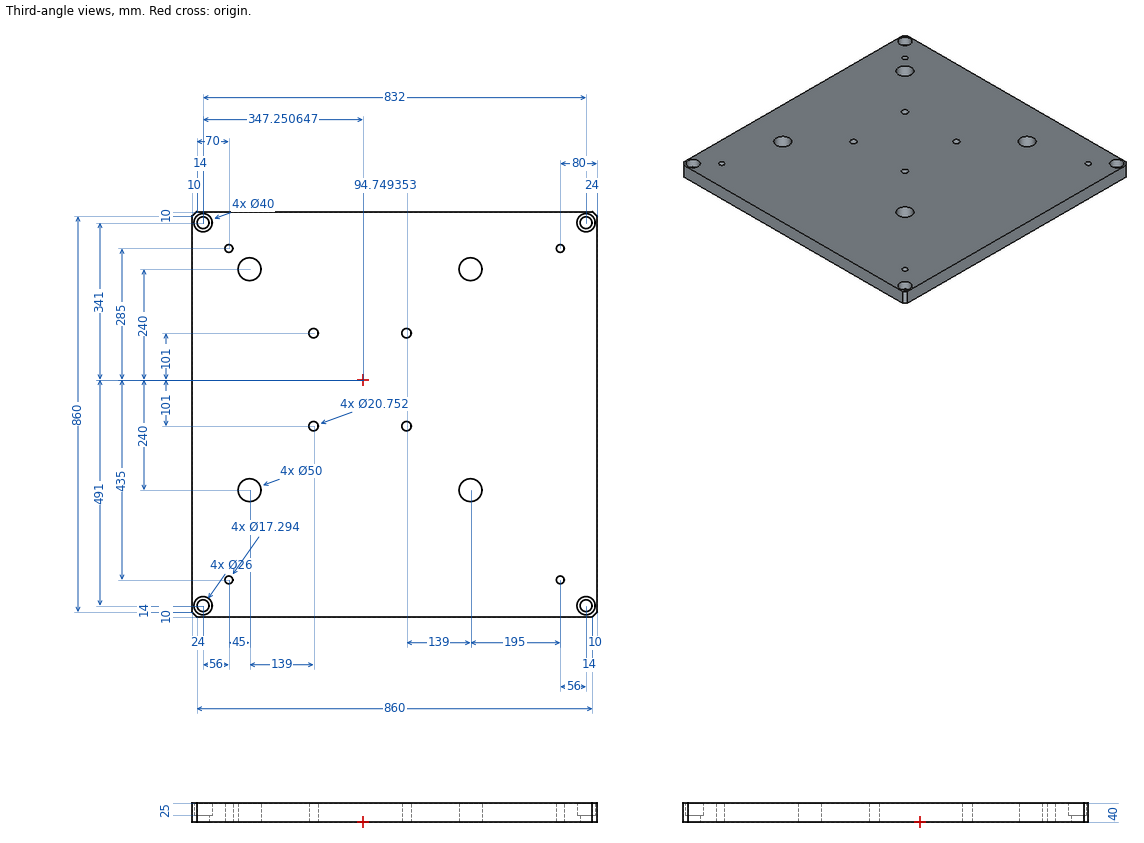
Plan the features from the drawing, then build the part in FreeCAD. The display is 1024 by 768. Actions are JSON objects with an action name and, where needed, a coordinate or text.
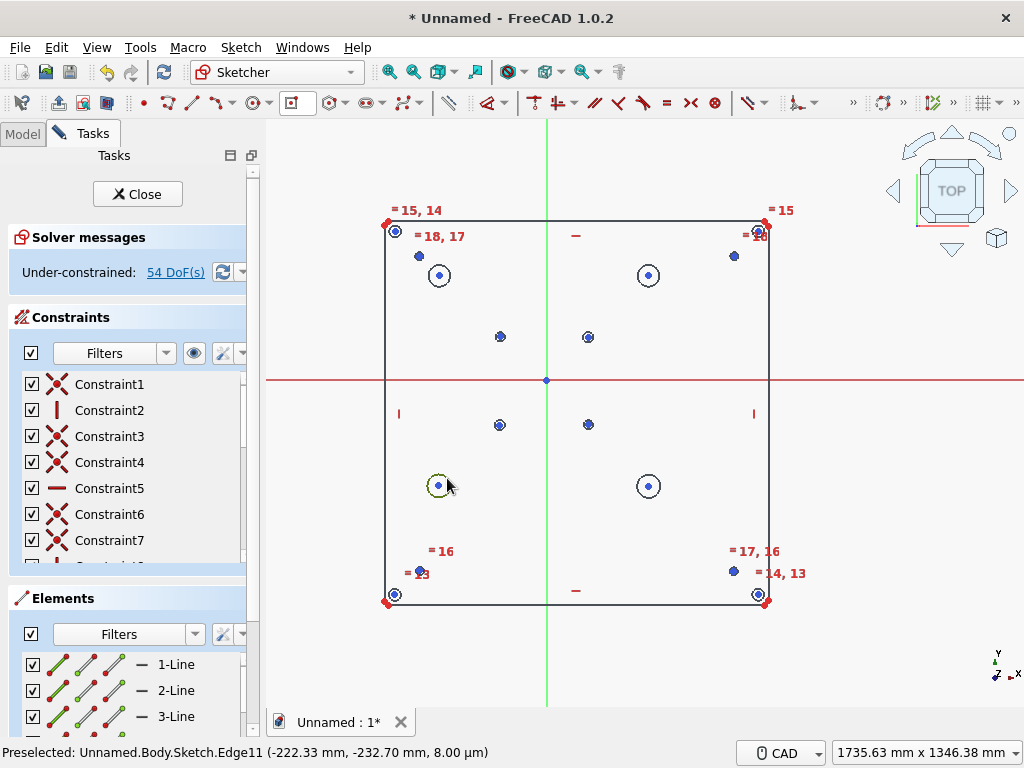
{"action": "left_click", "coordinate": [657, 478]}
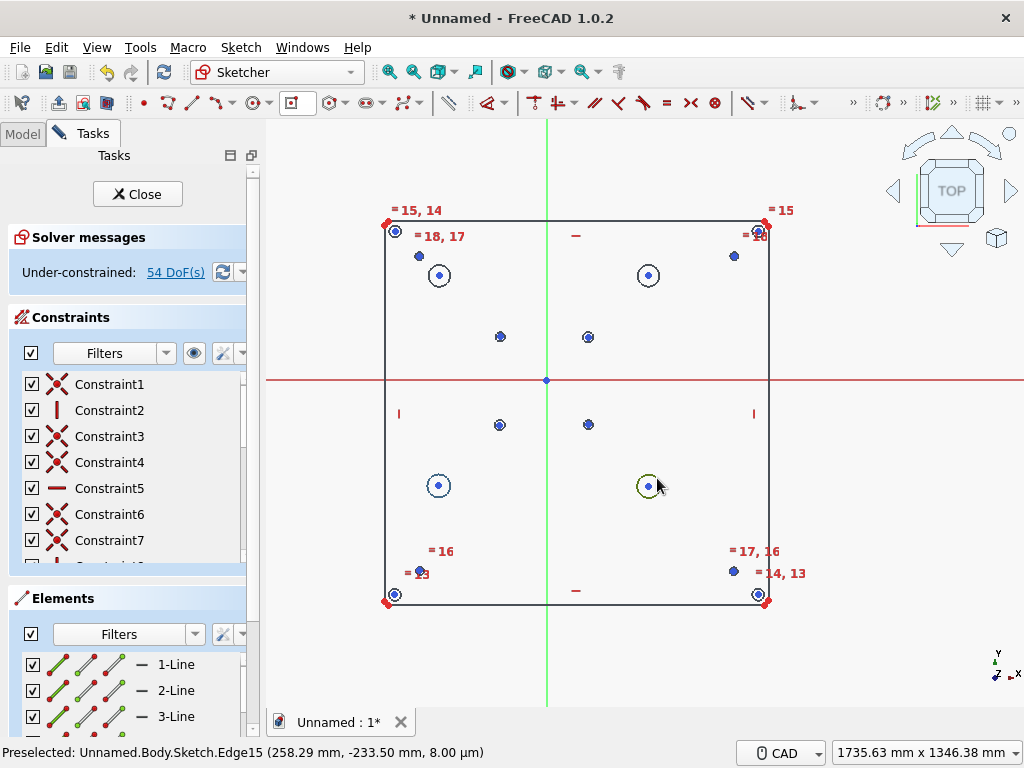
{"action": "scroll", "coordinate": [447, 268], "scroll_direction": "up", "scroll_amount": 2}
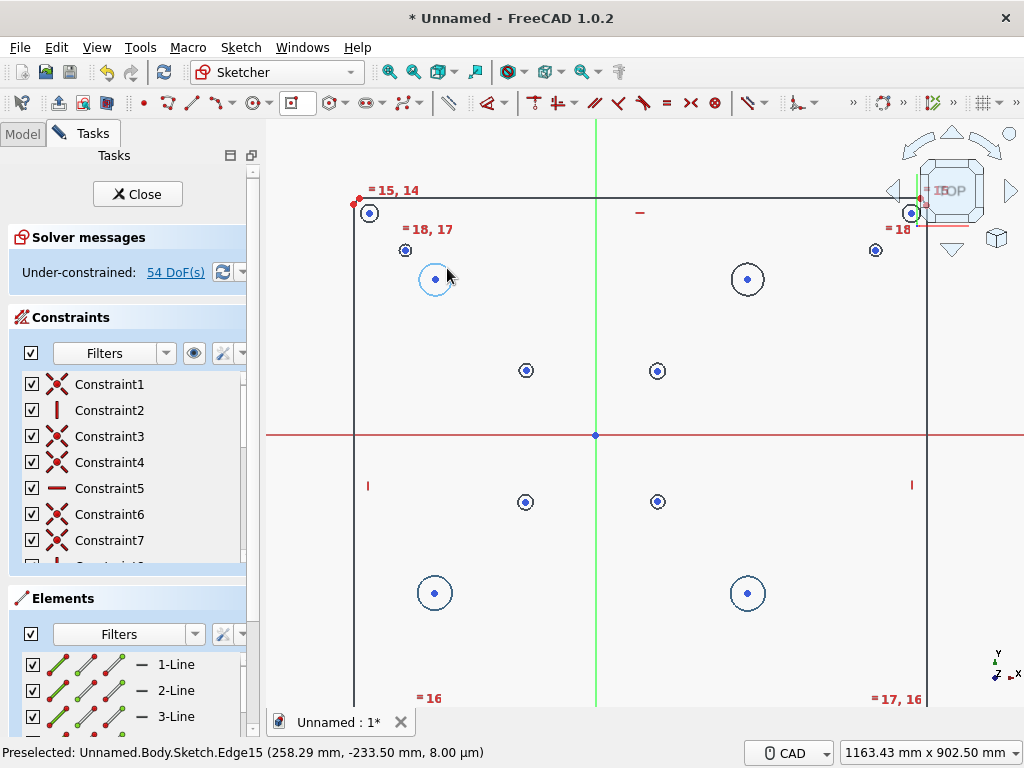
{"action": "left_click", "coordinate": [447, 268]}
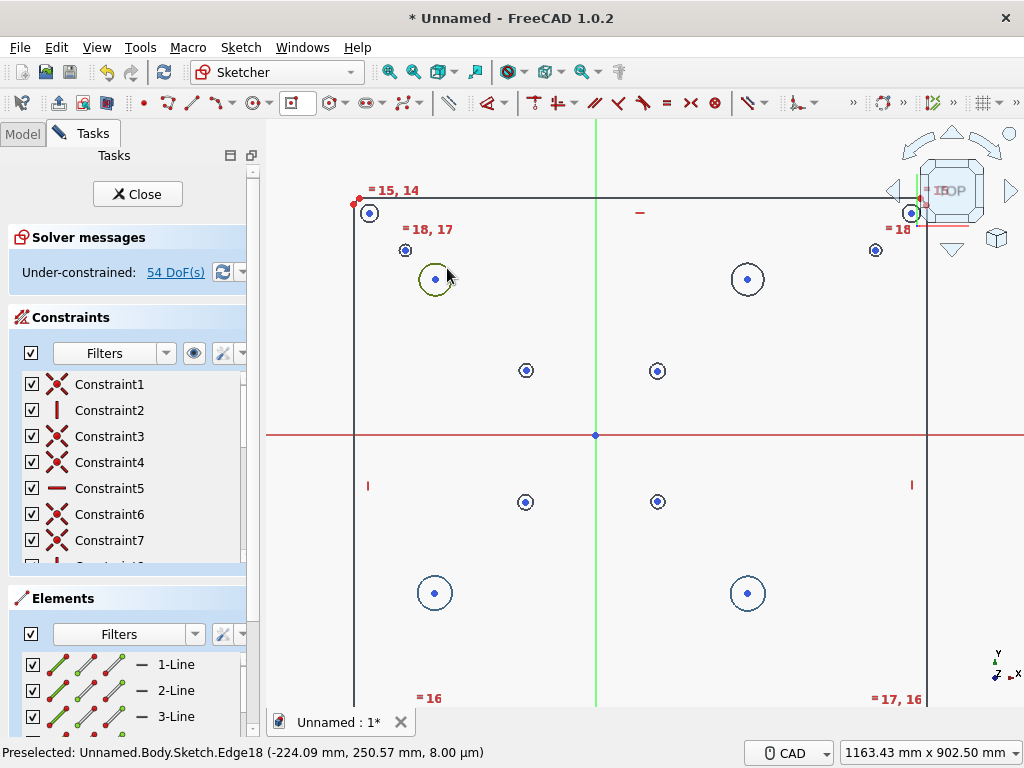
{"action": "left_click", "coordinate": [759, 268]}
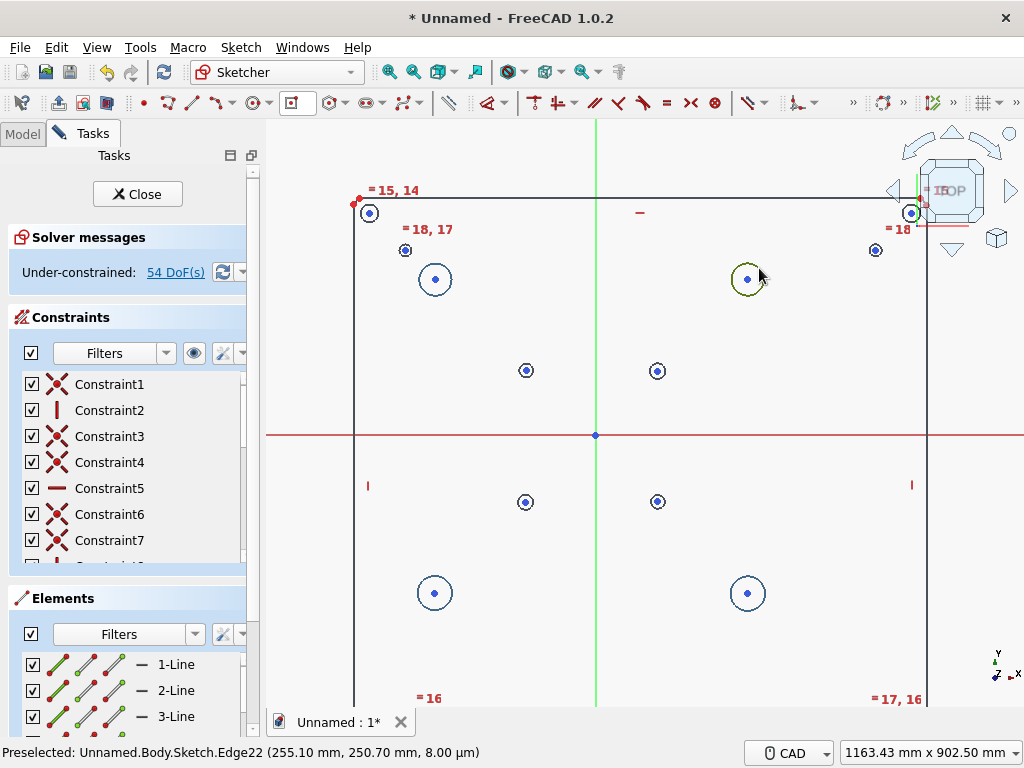
{"action": "left_click", "coordinate": [668, 104]}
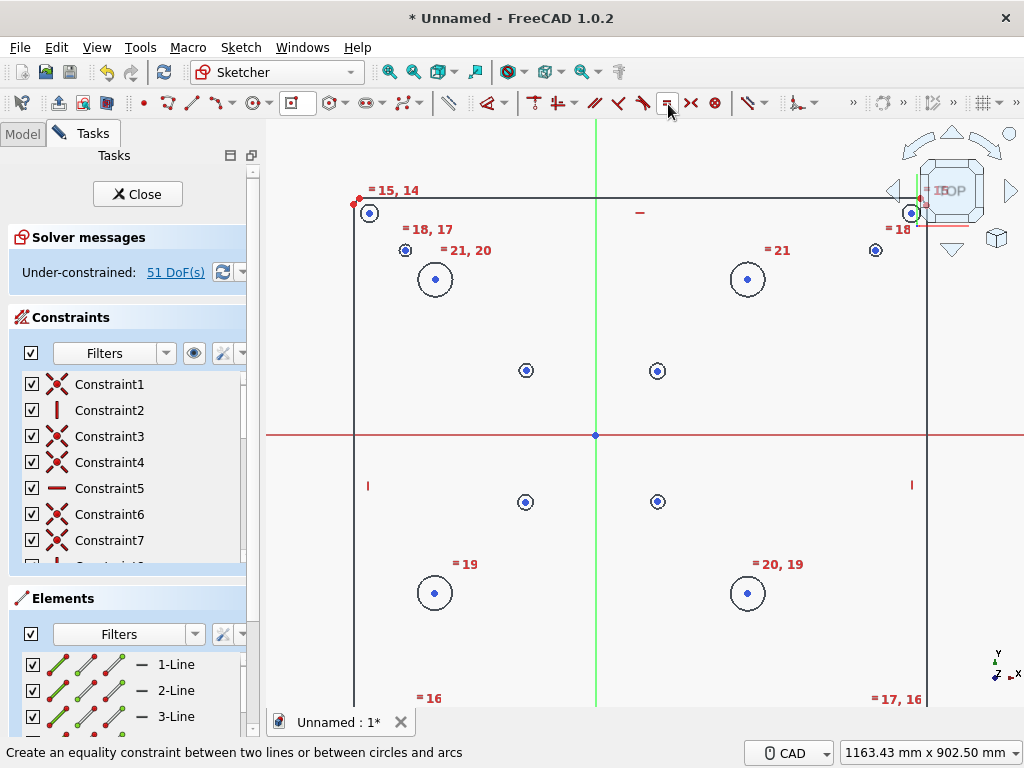
{"action": "scroll", "coordinate": [531, 508], "scroll_direction": "up", "scroll_amount": 4}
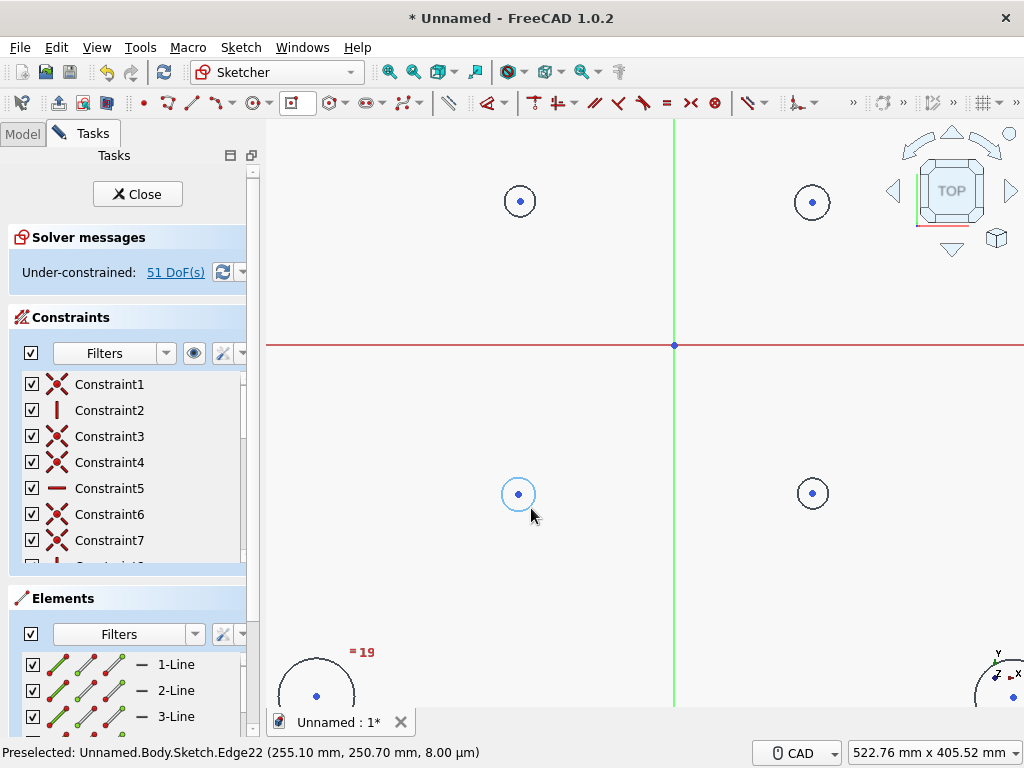
{"action": "left_click", "coordinate": [530, 506]}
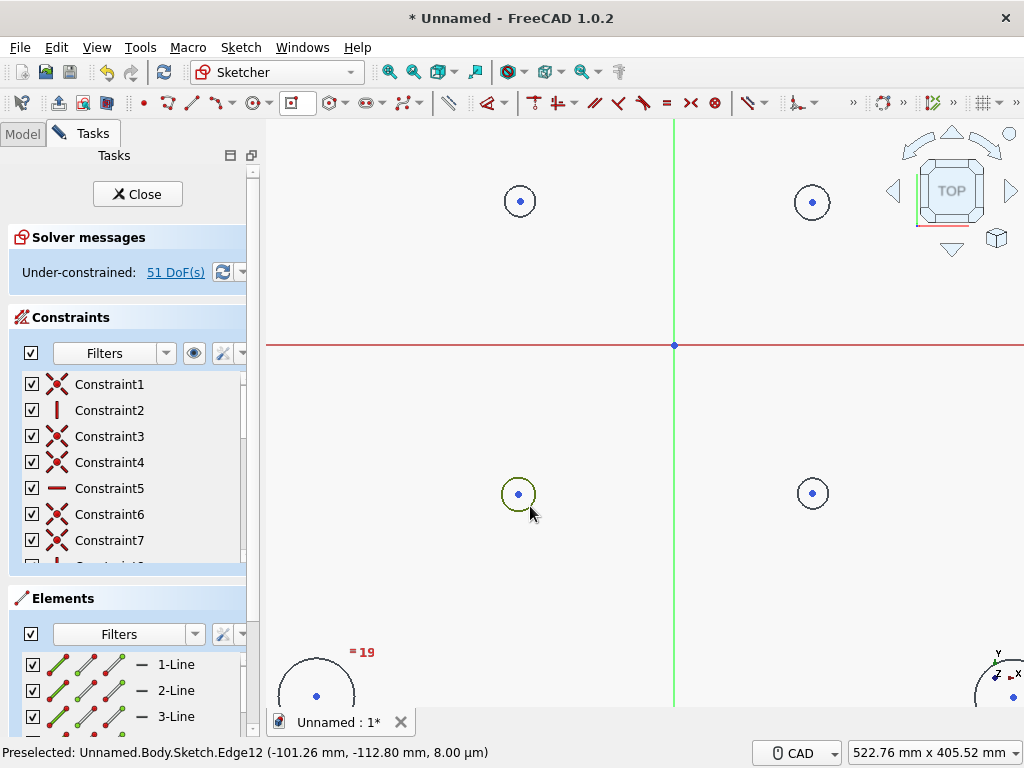
{"action": "left_click", "coordinate": [824, 483]}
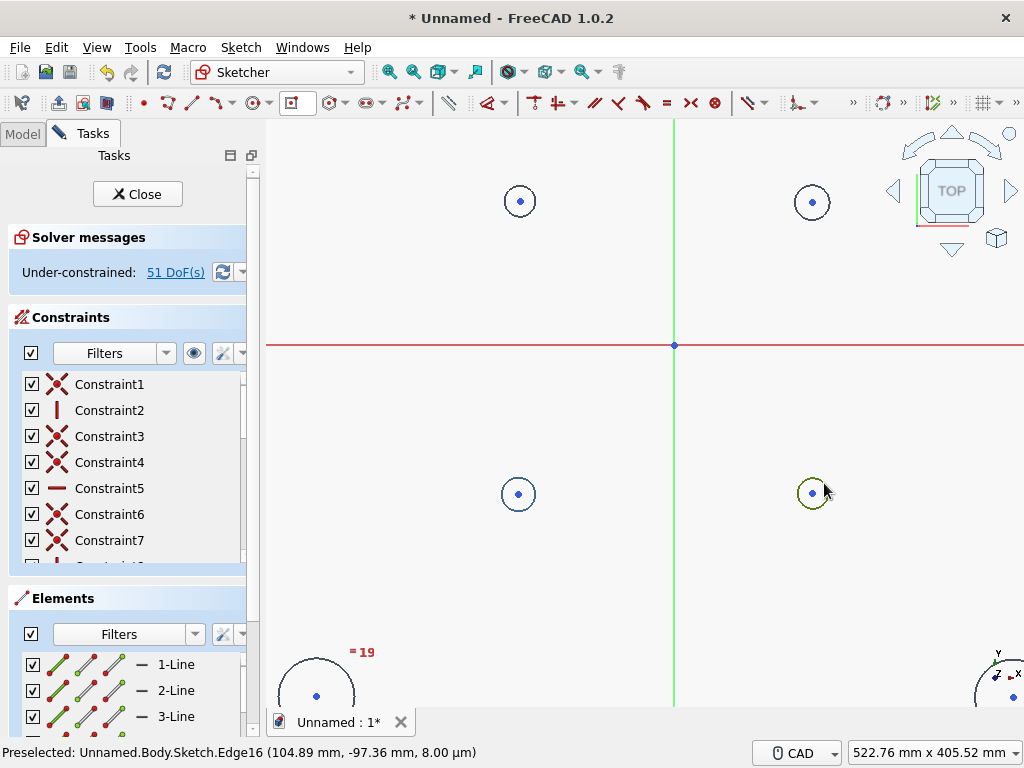
{"action": "left_click", "coordinate": [531, 190]}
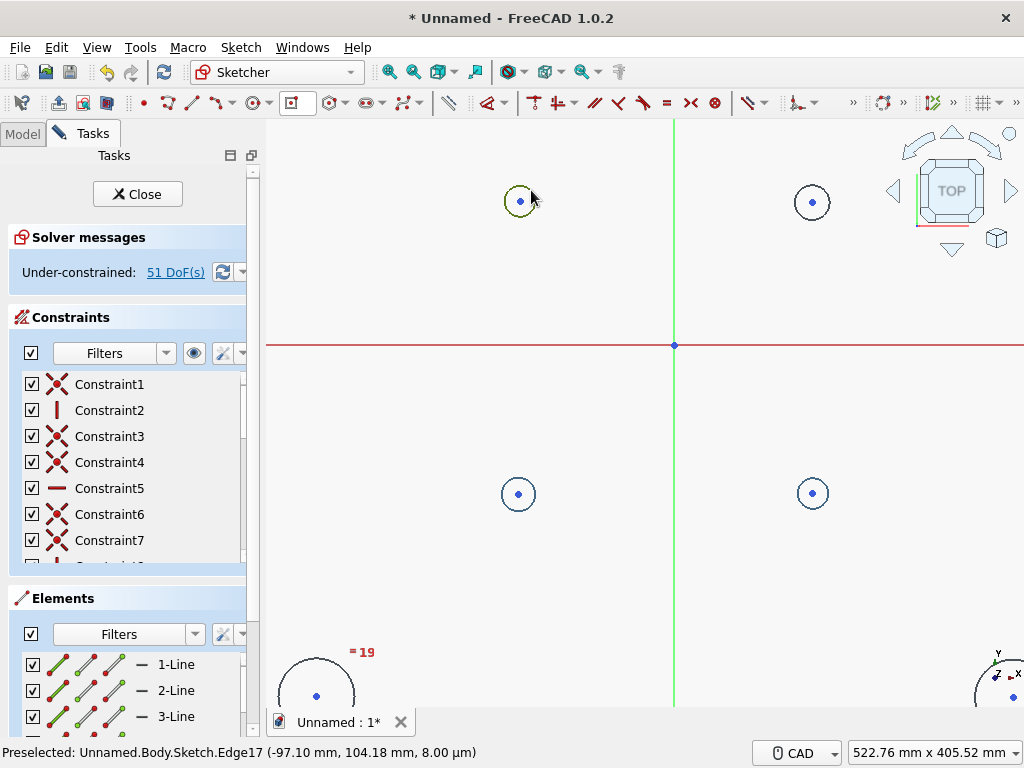
{"action": "left_click", "coordinate": [824, 190]}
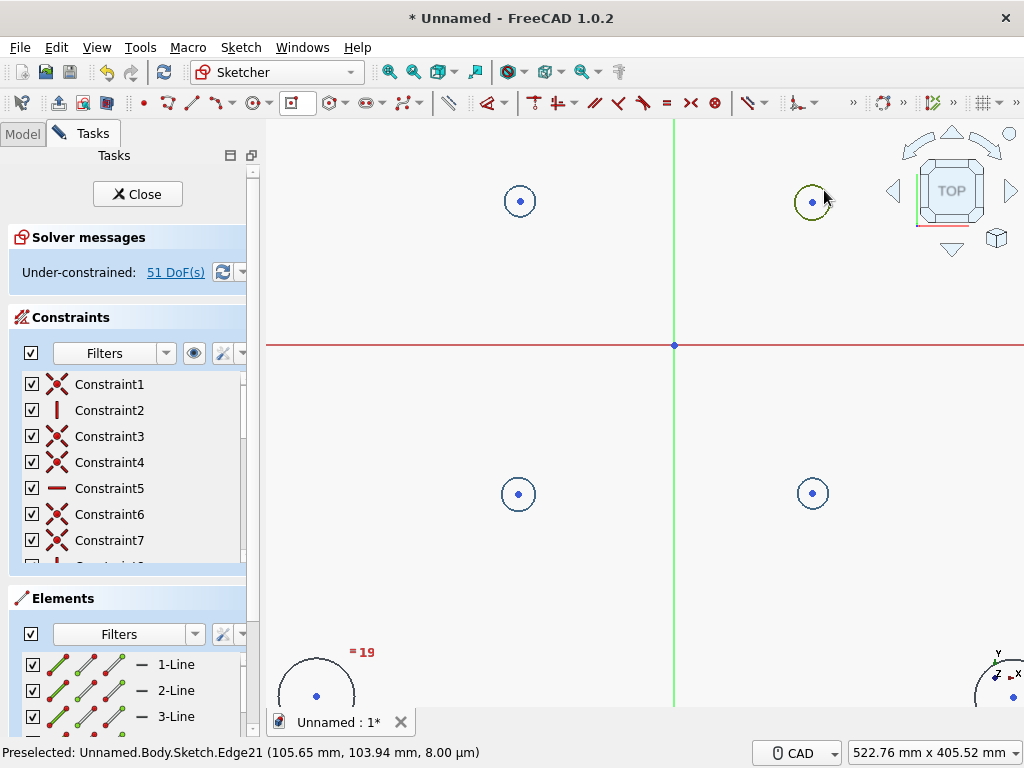
{"action": "key", "text": "e"}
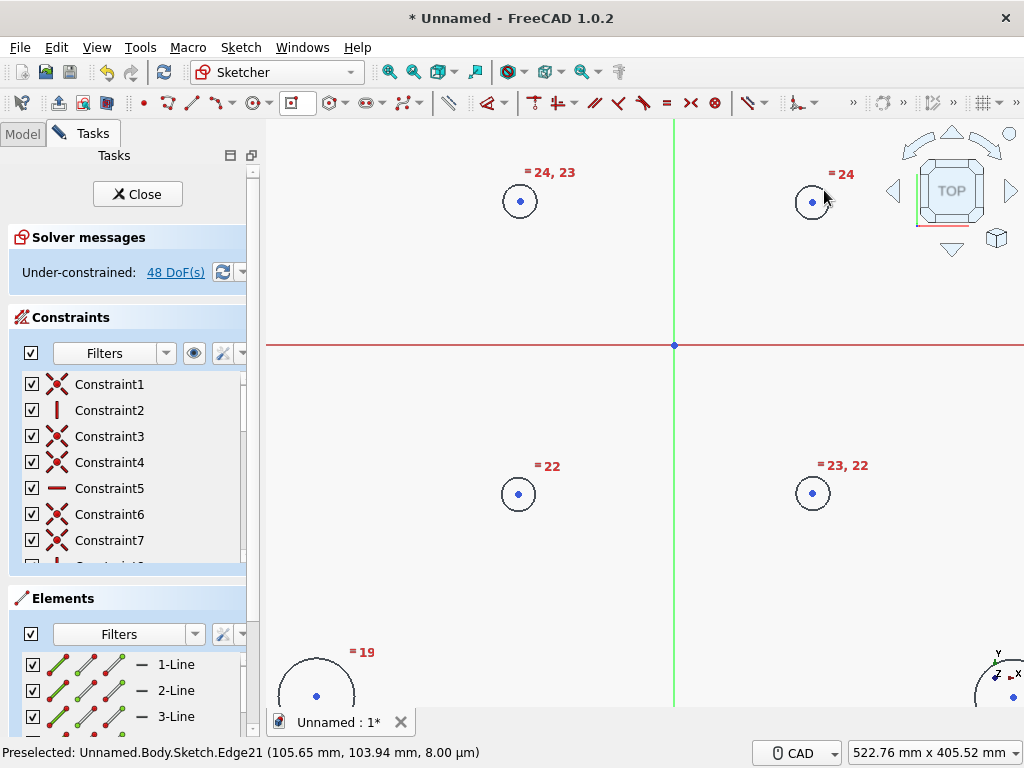
{"action": "left_click", "coordinate": [518, 494]}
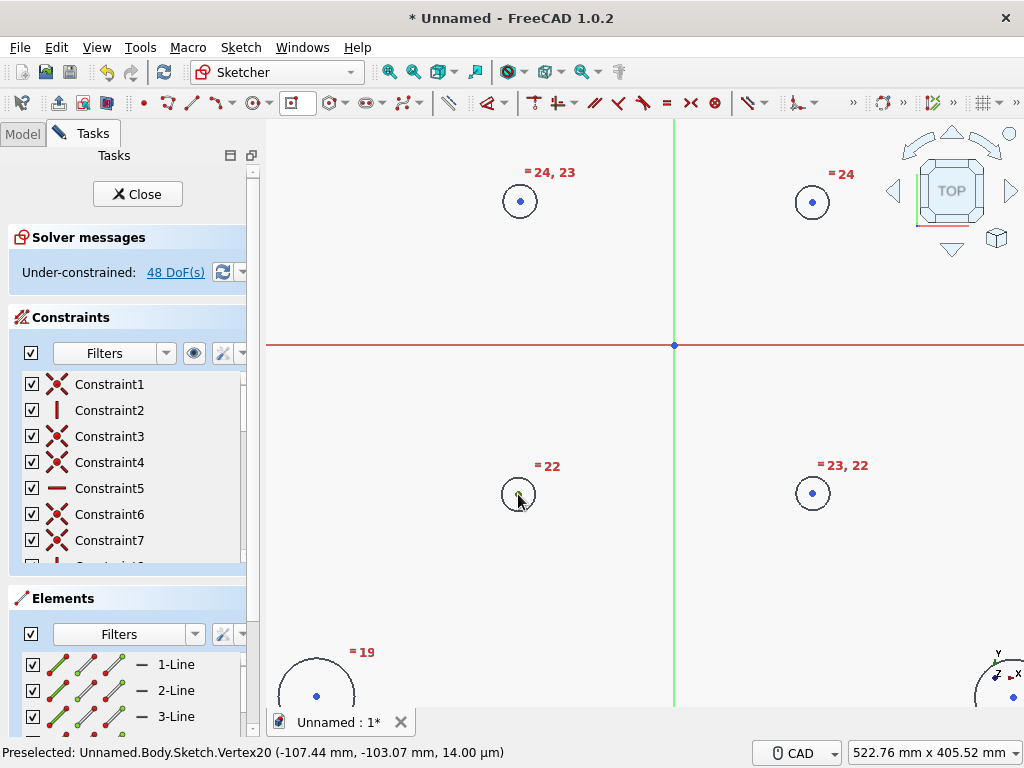
{"action": "left_click", "coordinate": [813, 494]}